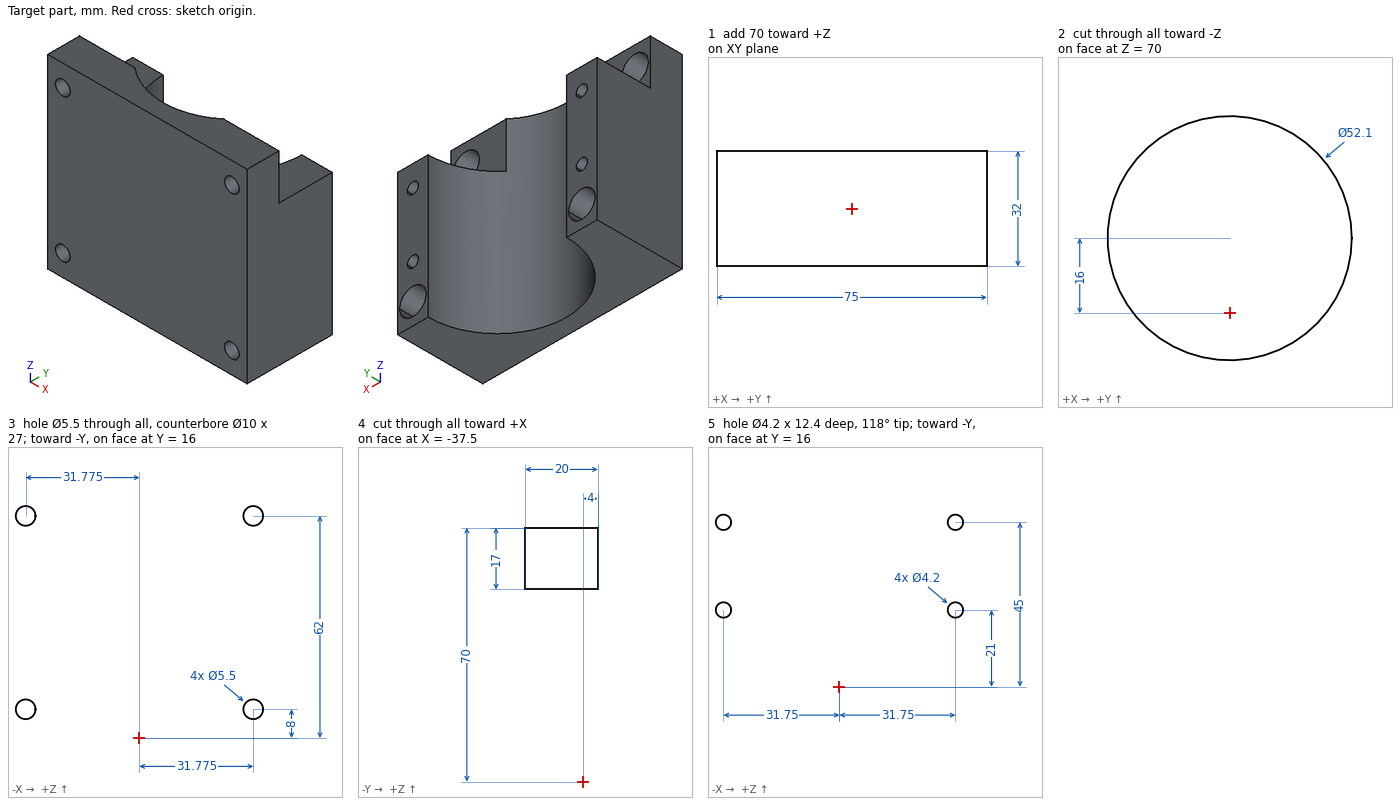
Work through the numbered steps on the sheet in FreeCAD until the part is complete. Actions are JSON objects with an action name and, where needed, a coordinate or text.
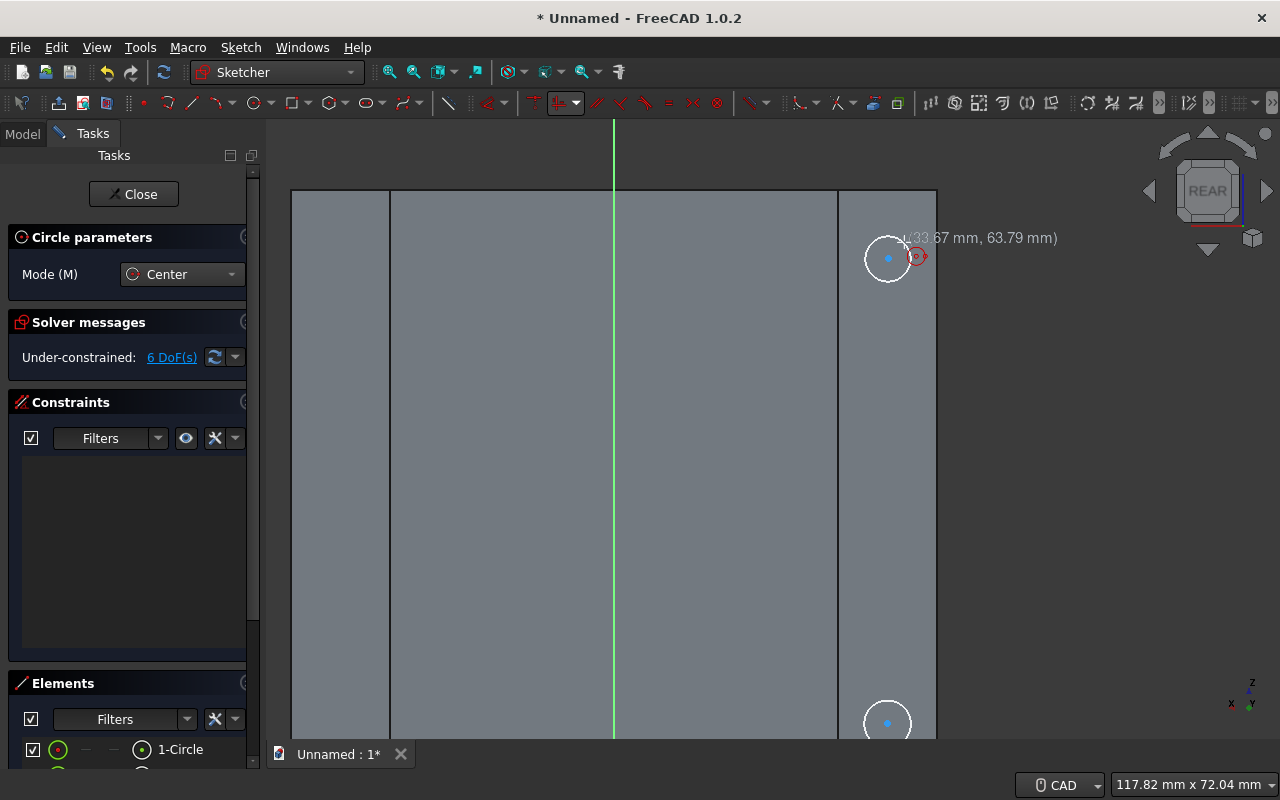
{"action": "left_click", "coordinate": [341, 258]}
{"action": "left_click", "coordinate": [357, 242]}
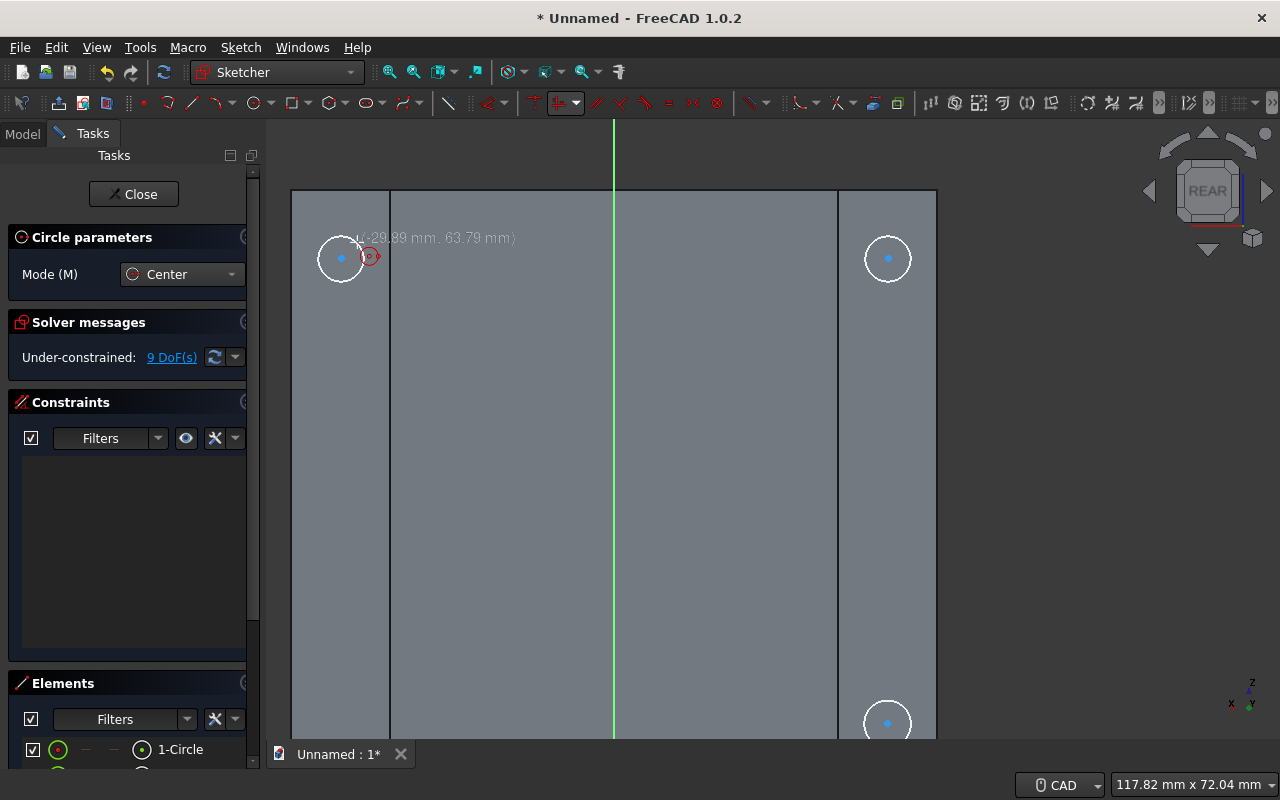
{"action": "scroll", "coordinate": [888, 257], "scroll_direction": "down", "scroll_amount": 2}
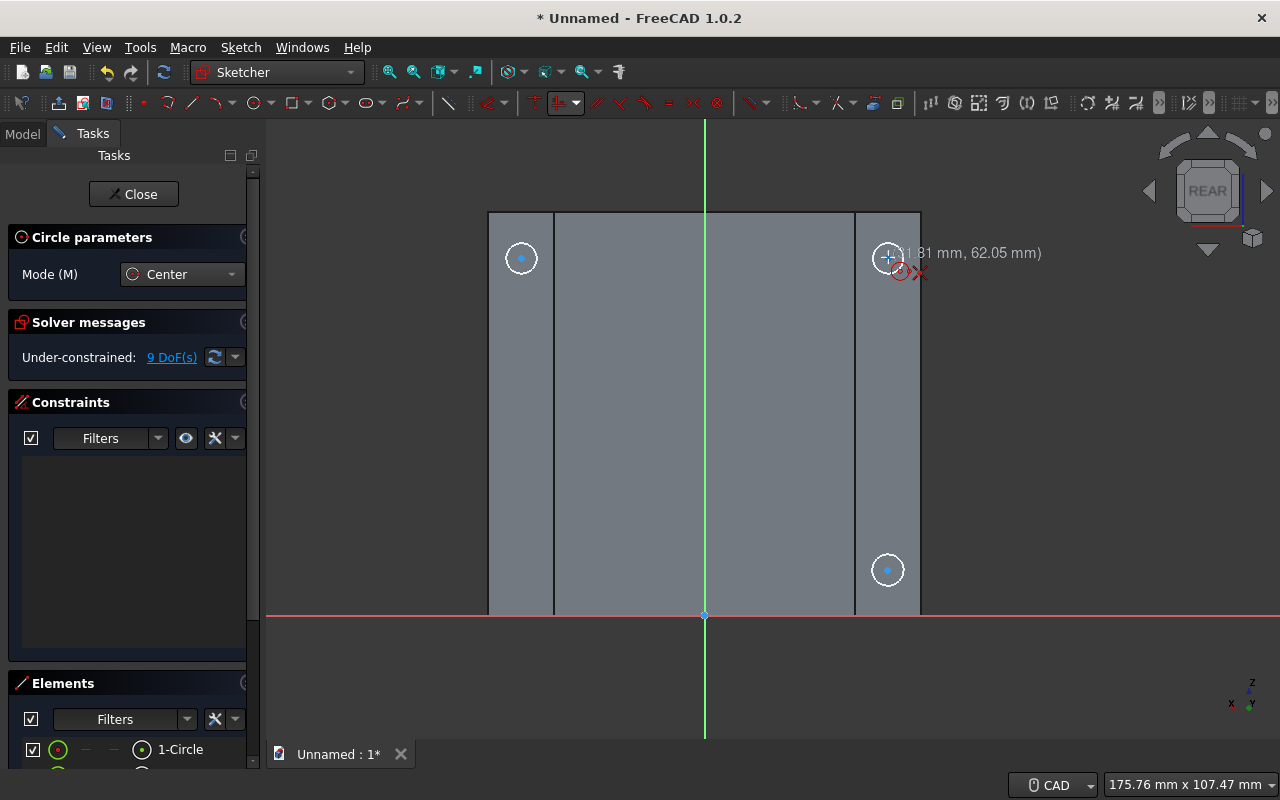
{"action": "scroll", "coordinate": [521, 570], "scroll_direction": "up", "scroll_amount": 2}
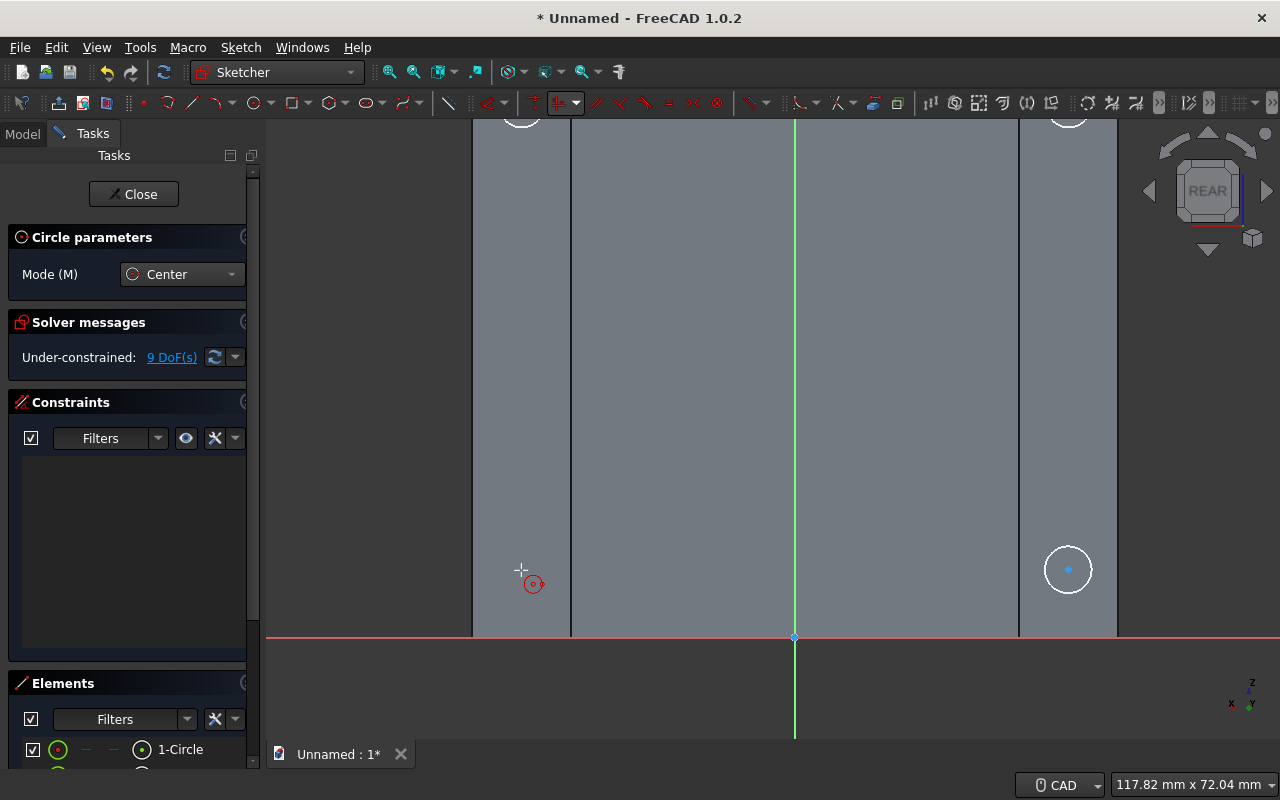
{"action": "left_click", "coordinate": [521, 569]}
{"action": "left_click", "coordinate": [538, 552]}
{"action": "key", "text": "Escape"}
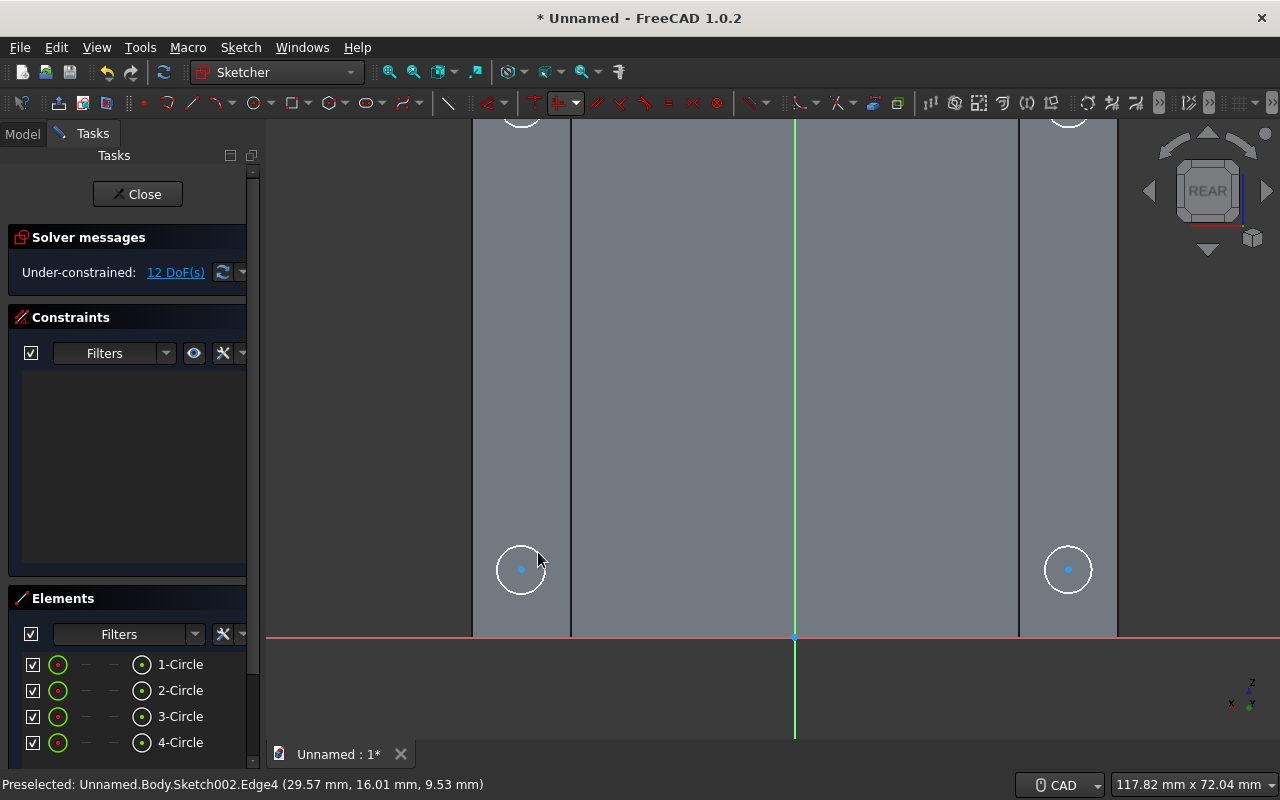
{"action": "left_click", "coordinate": [1085, 553]}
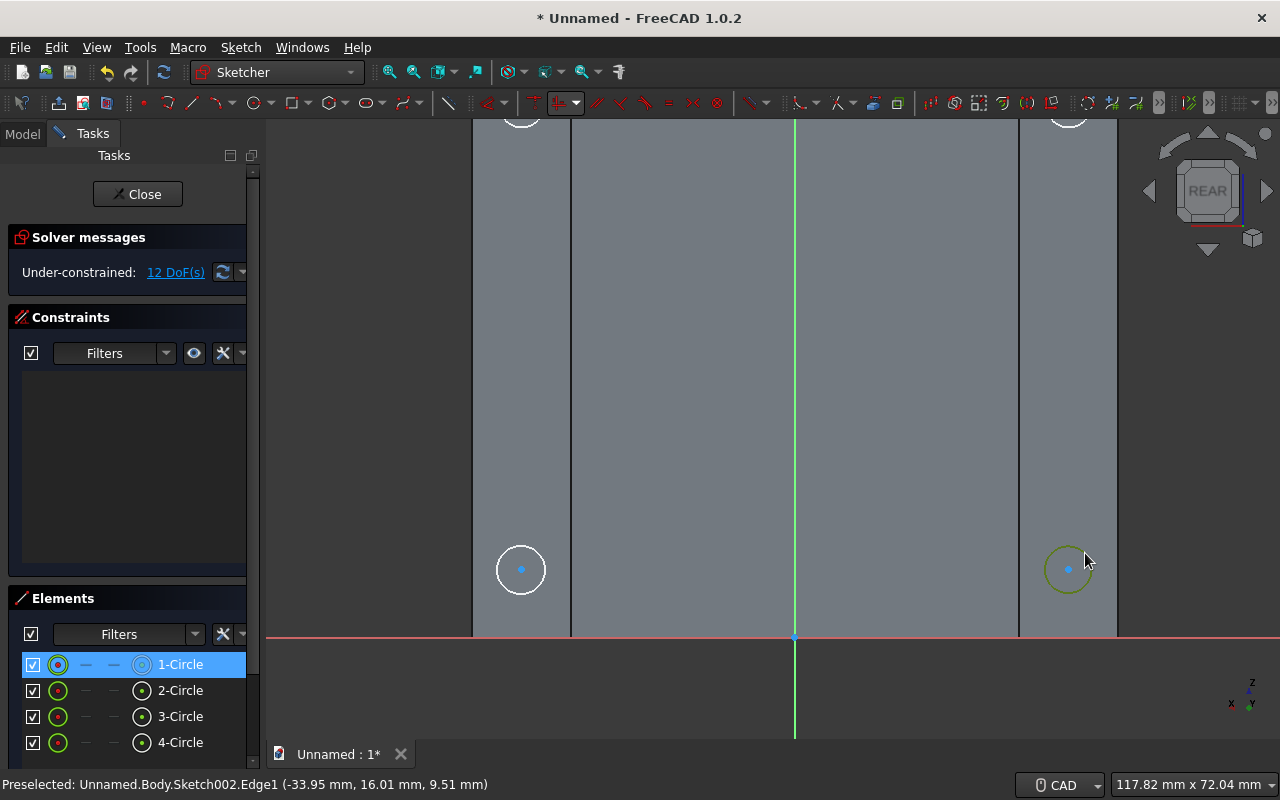
{"action": "scroll", "coordinate": [521, 571], "scroll_direction": "down", "scroll_amount": 2}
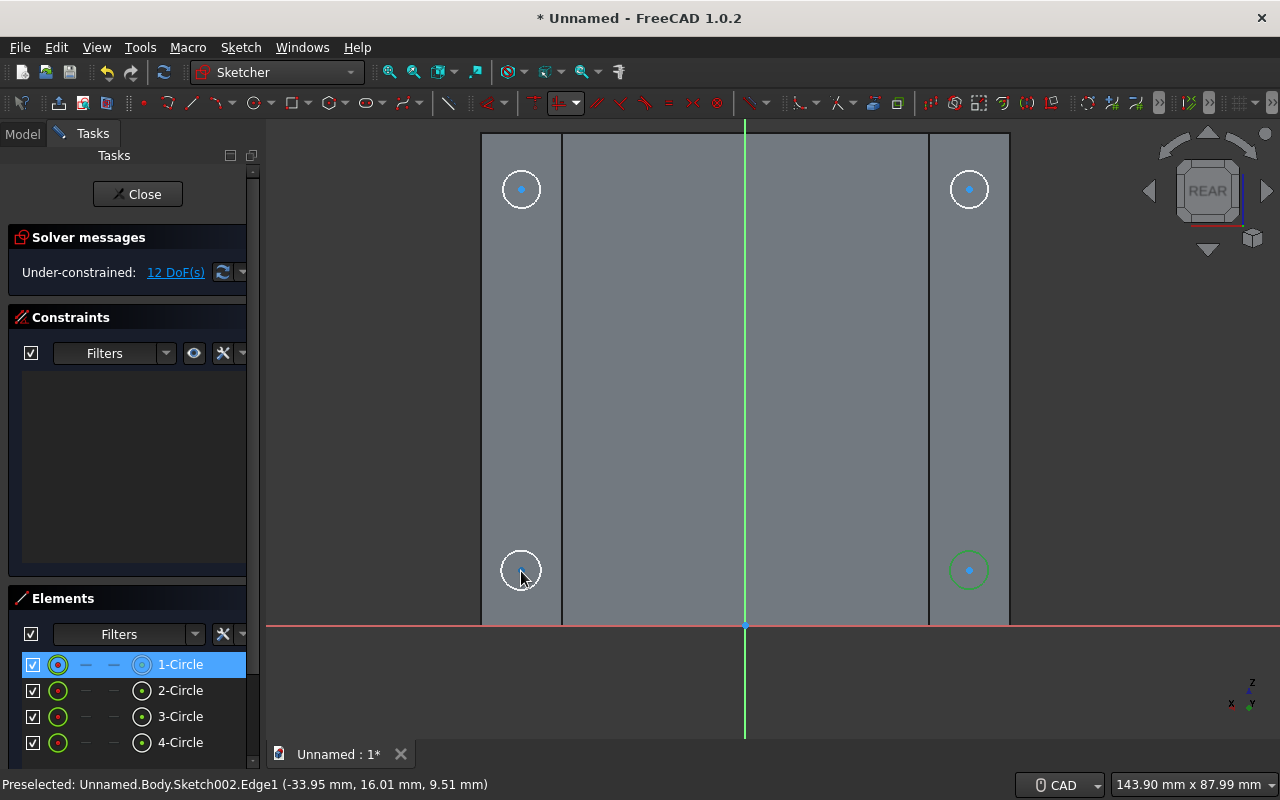
{"action": "left_click", "coordinate": [899, 248]}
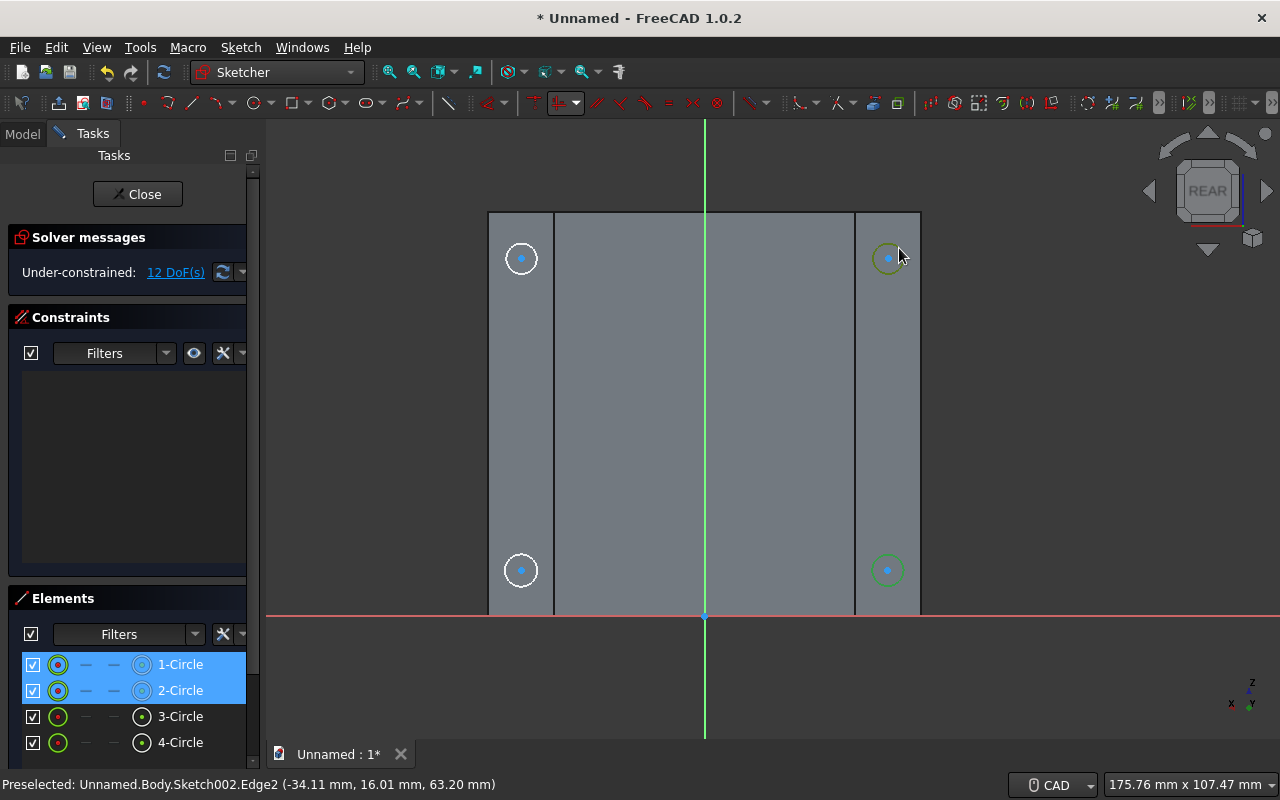
{"action": "left_click", "coordinate": [532, 248]}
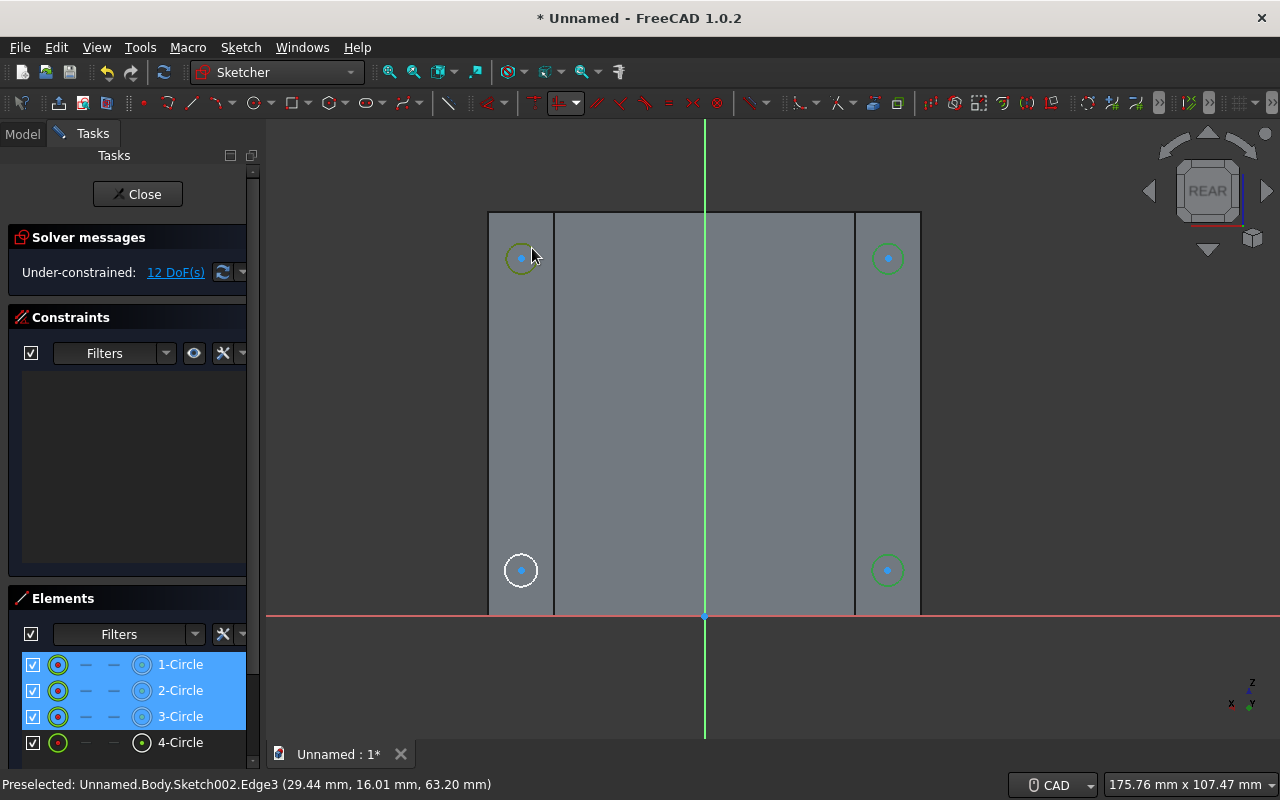
{"action": "left_click", "coordinate": [532, 559]}